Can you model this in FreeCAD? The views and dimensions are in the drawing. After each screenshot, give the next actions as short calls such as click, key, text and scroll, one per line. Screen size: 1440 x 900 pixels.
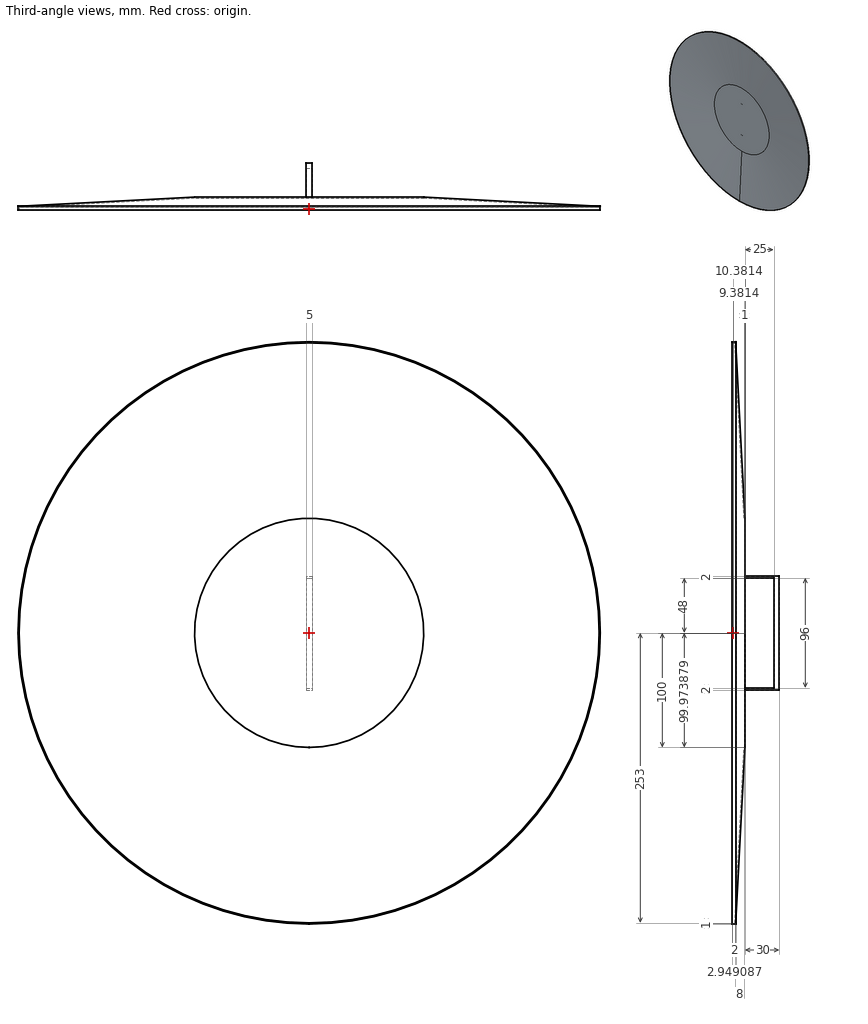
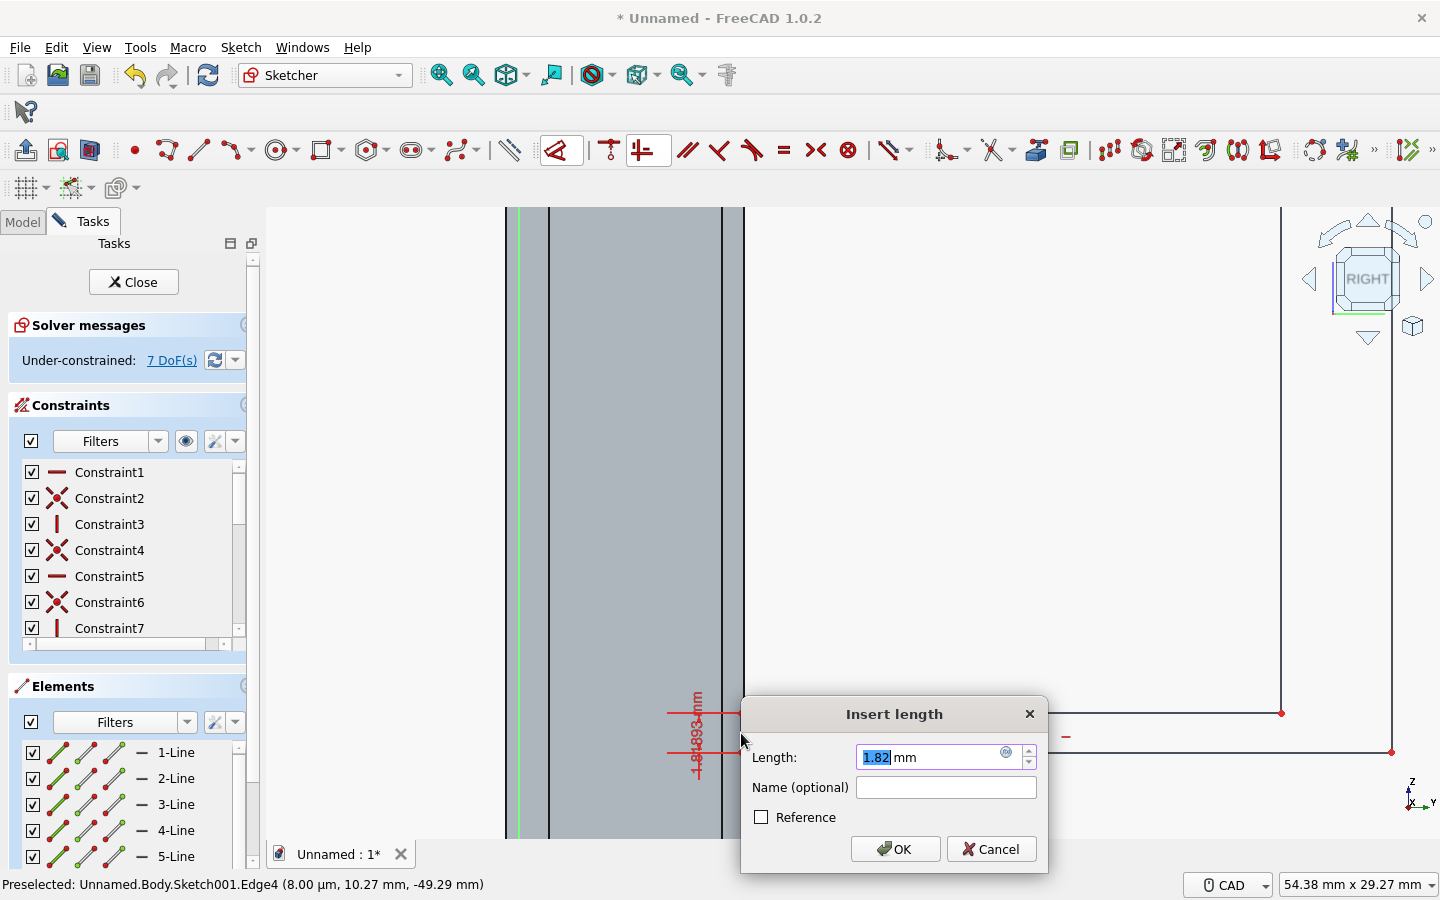
text(2)
key(Return)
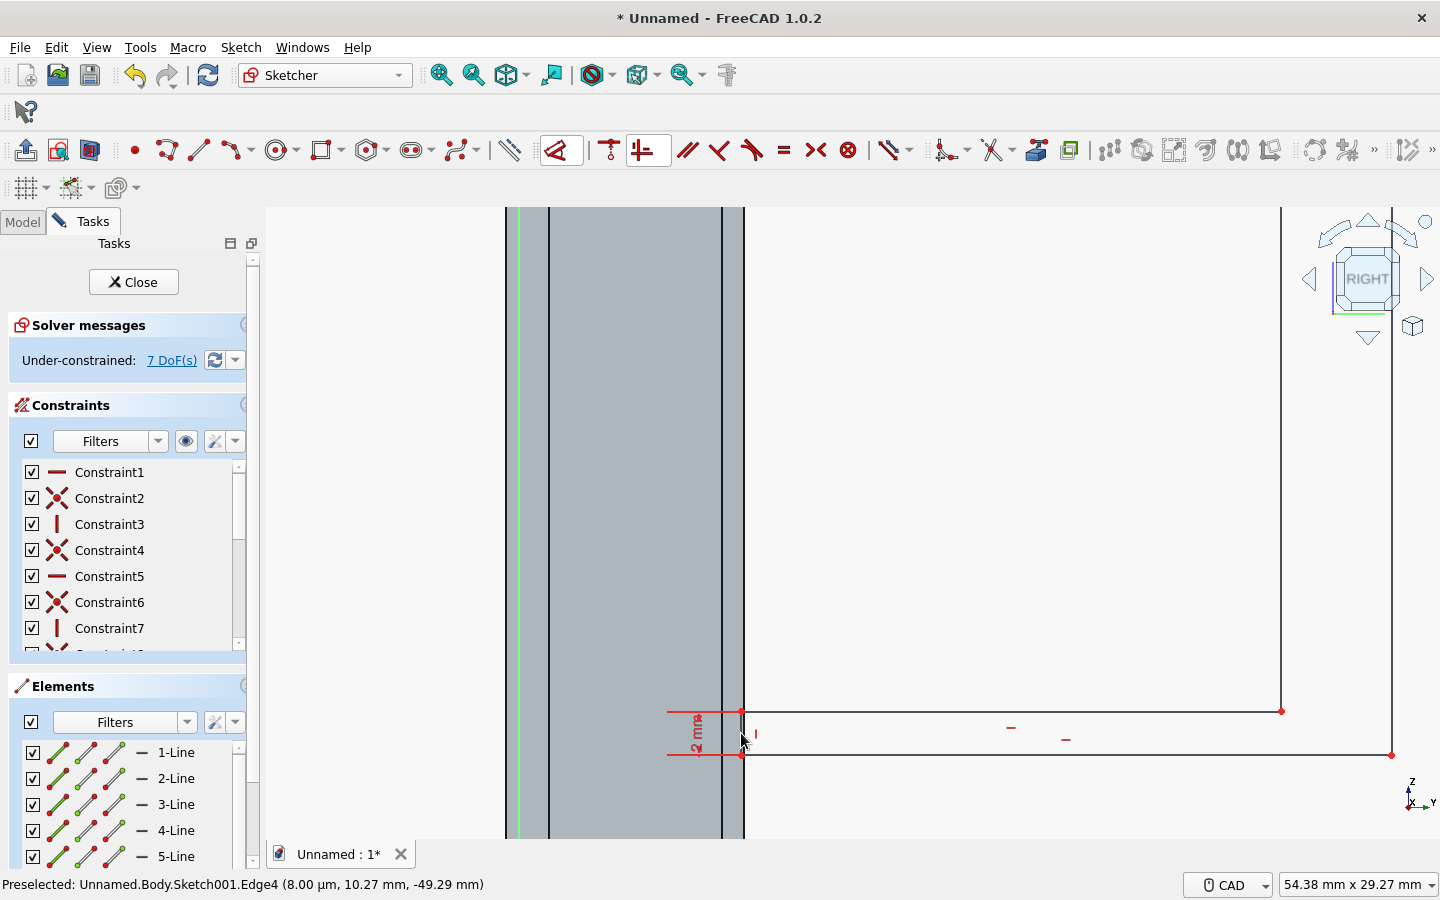
scroll(741, 739, down, 8)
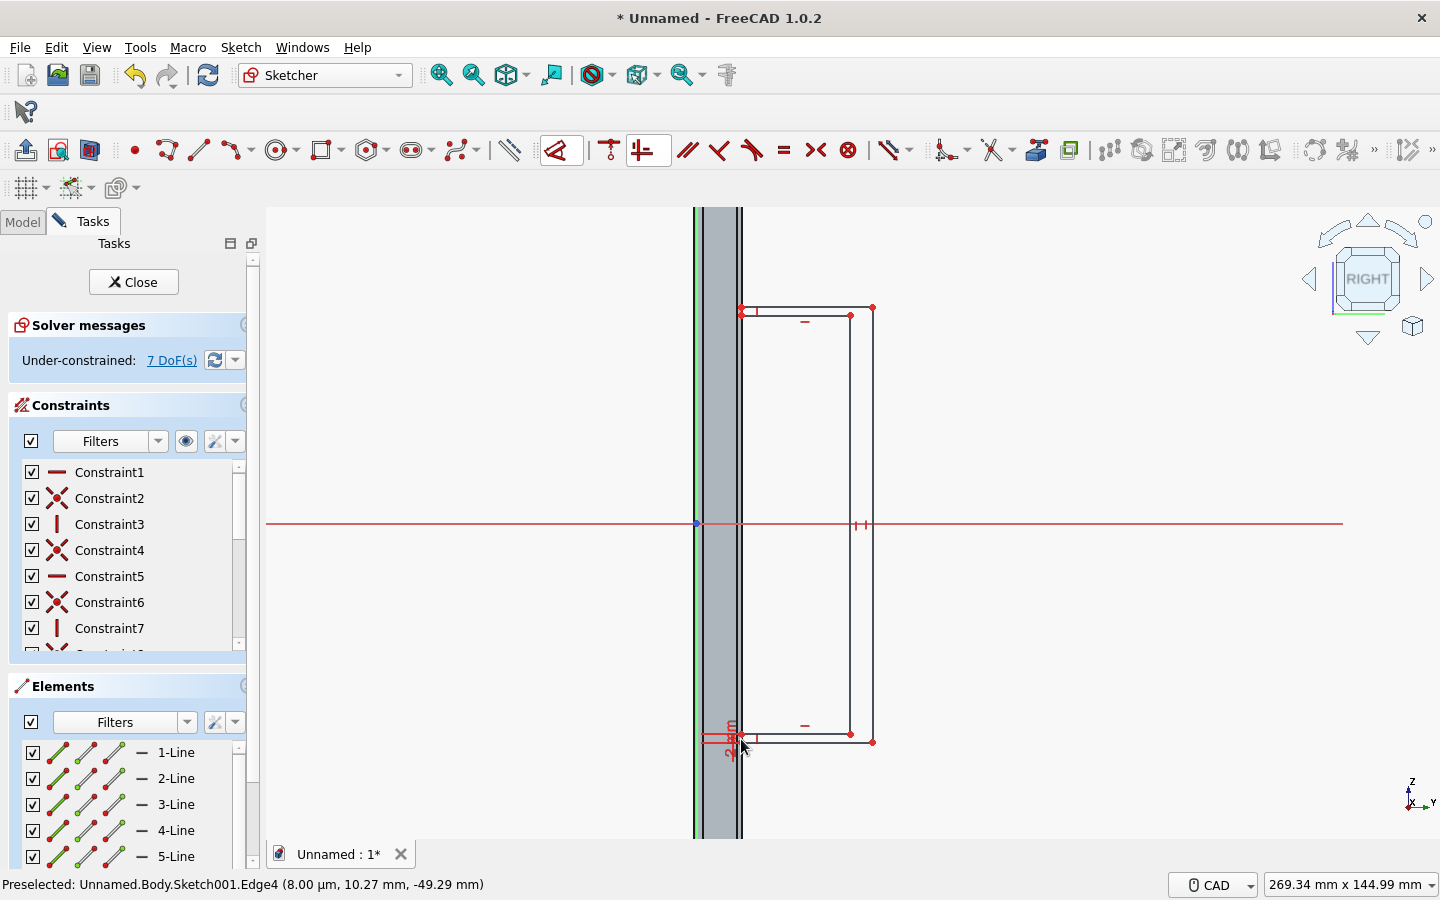
scroll(742, 310, up, 9)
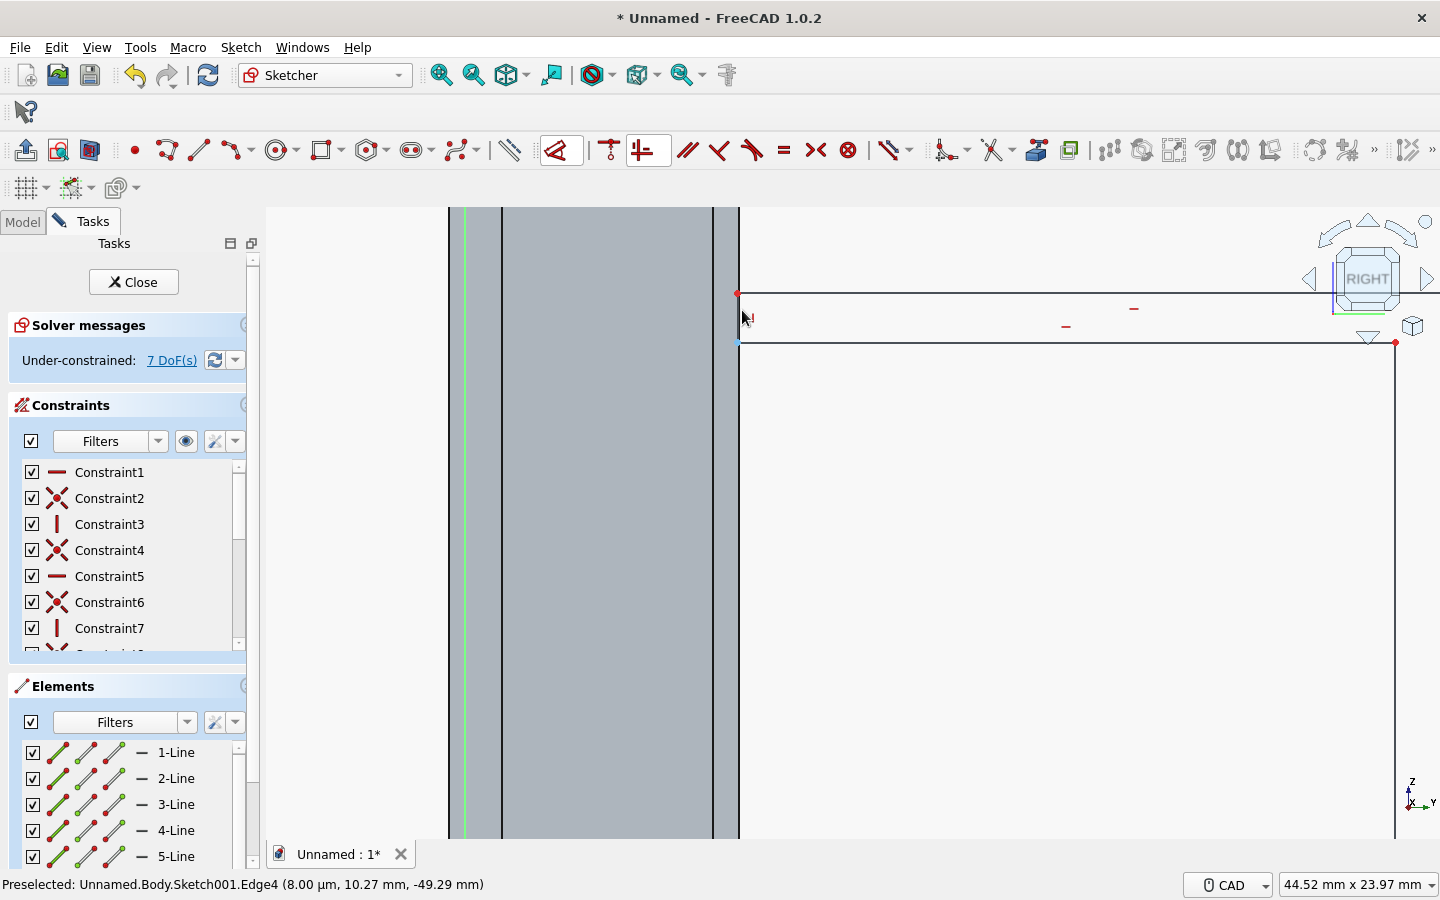
click(738, 308)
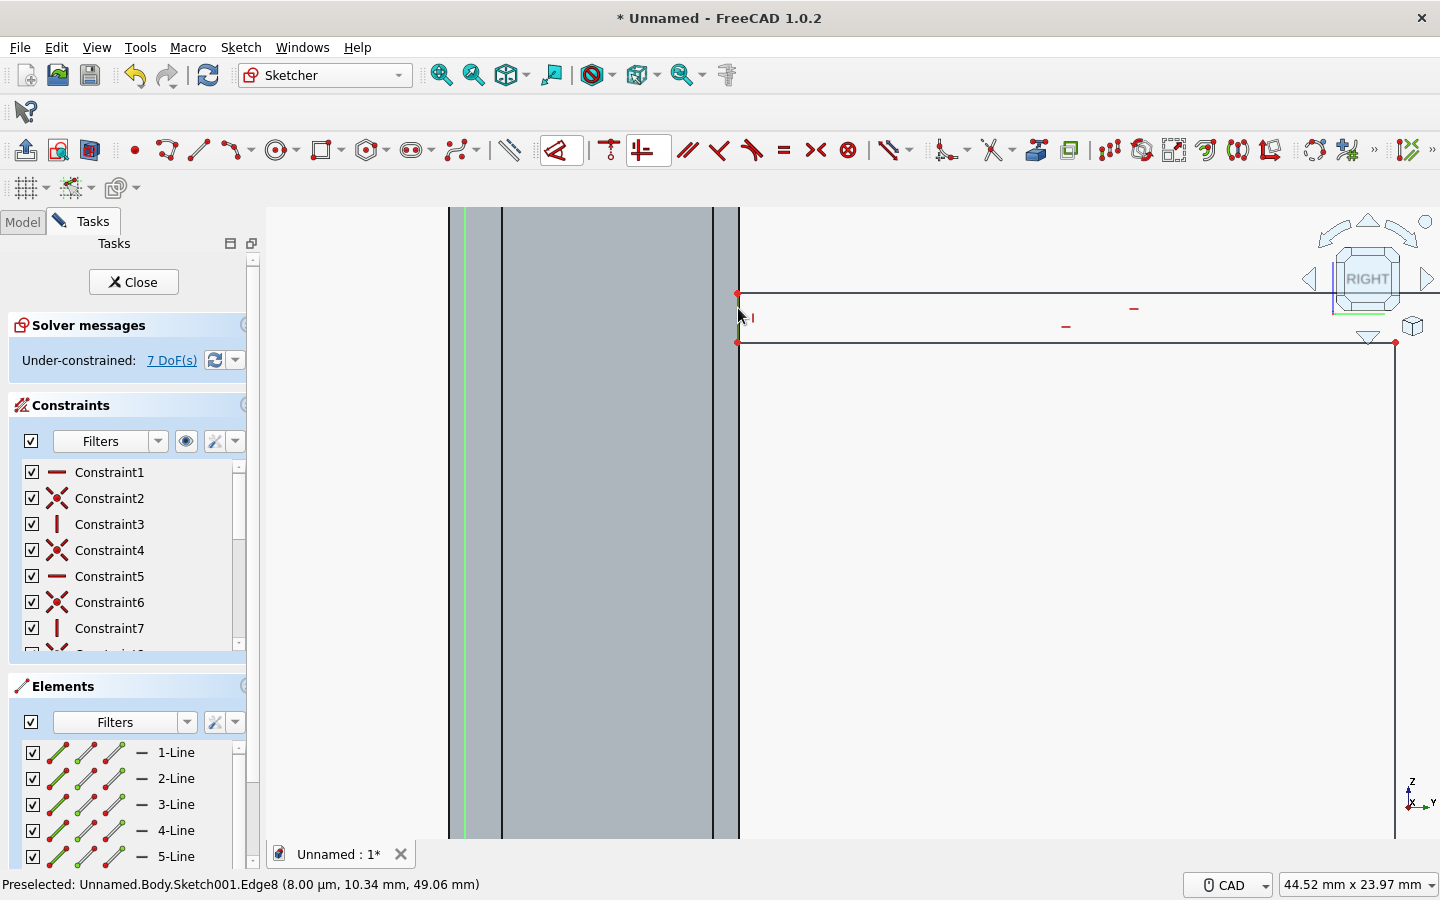
key(i)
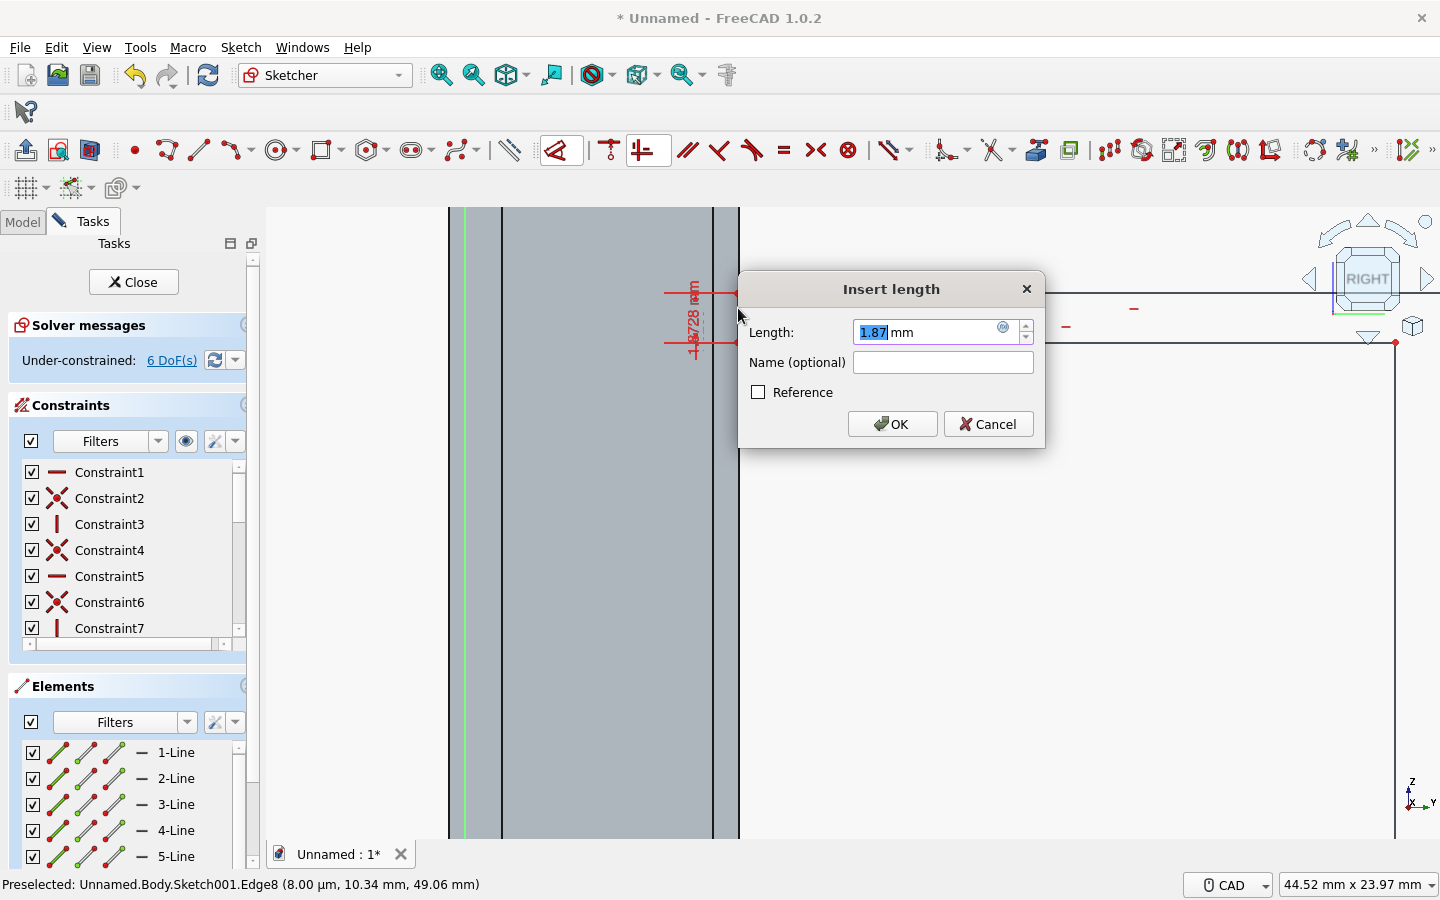
text(2)
key(Return)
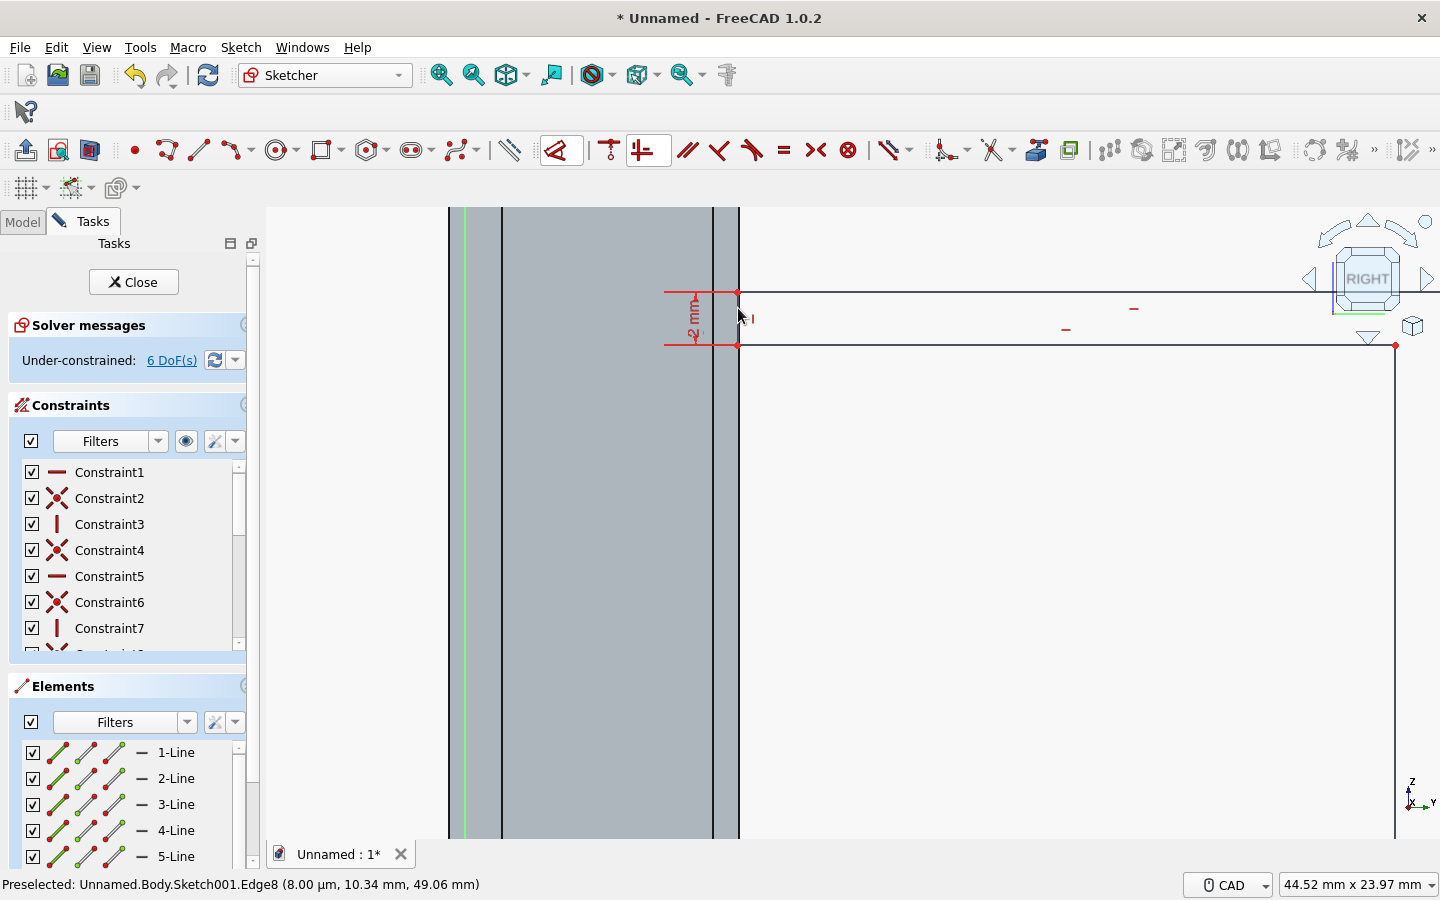
scroll(742, 309, down, 9)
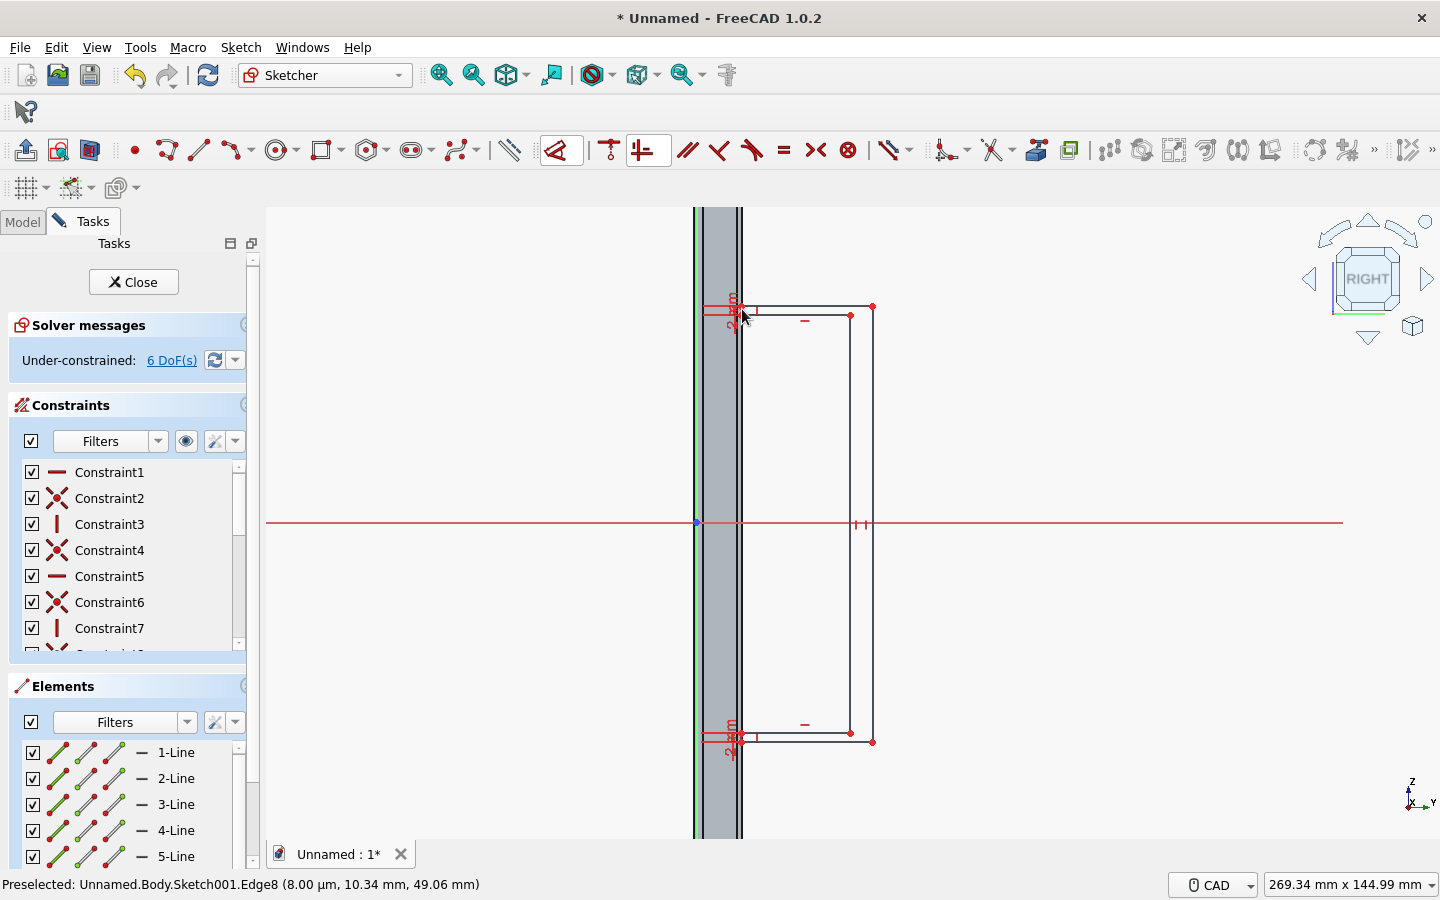
scroll(774, 315, up, 3)